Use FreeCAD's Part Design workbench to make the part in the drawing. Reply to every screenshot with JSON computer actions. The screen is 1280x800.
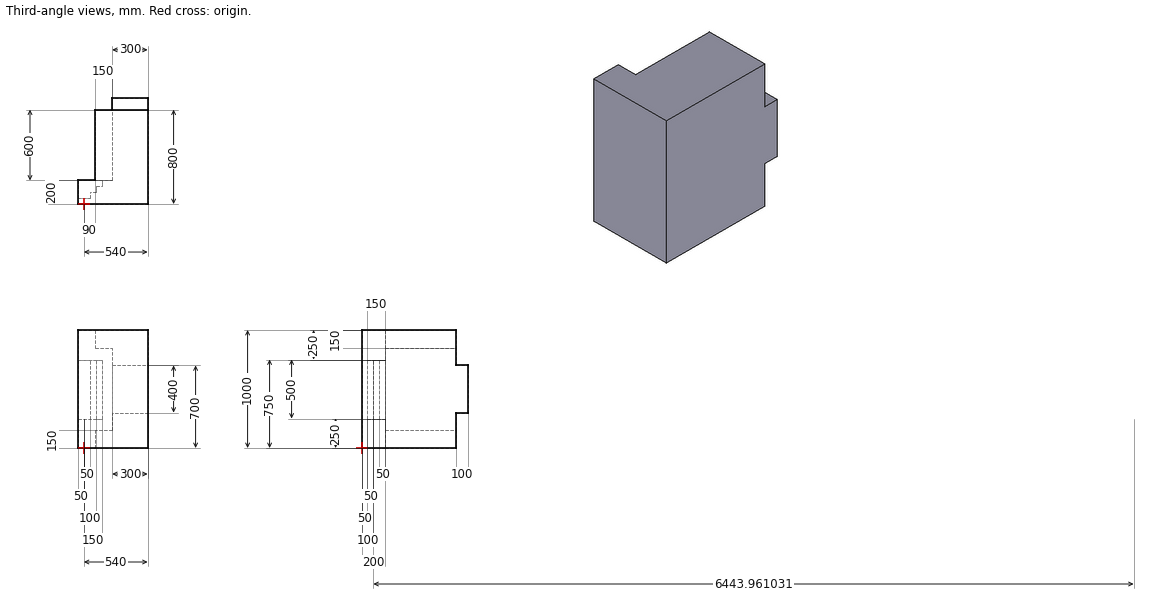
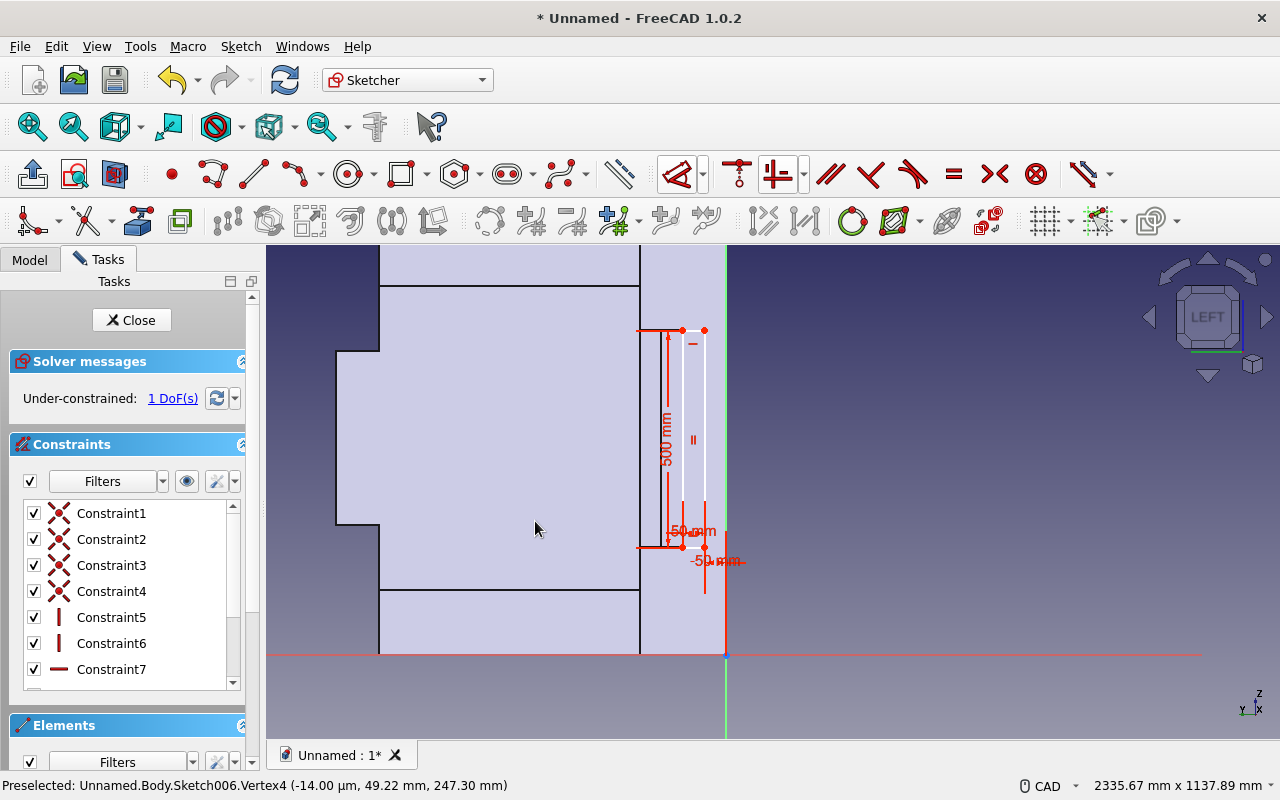
{"action": "left_click", "coordinate": [683, 331]}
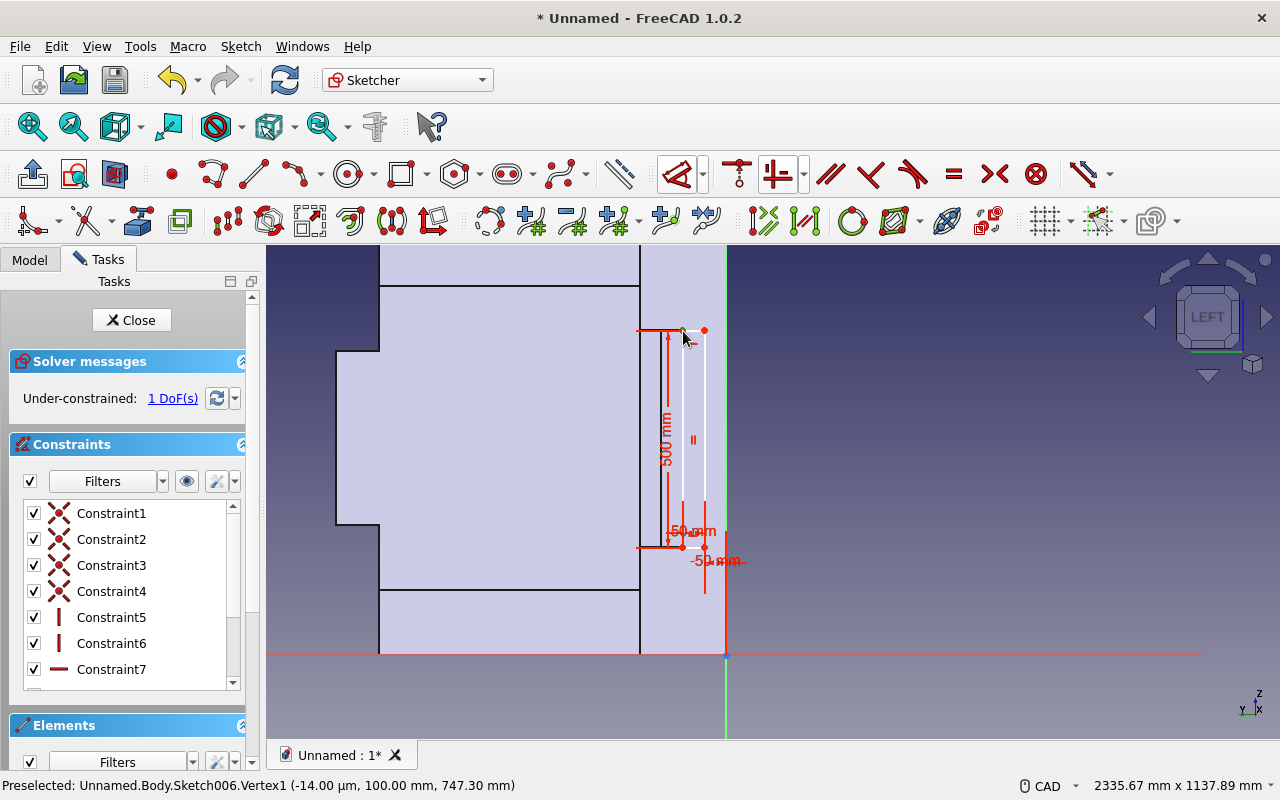
{"action": "left_click", "coordinate": [702, 174]}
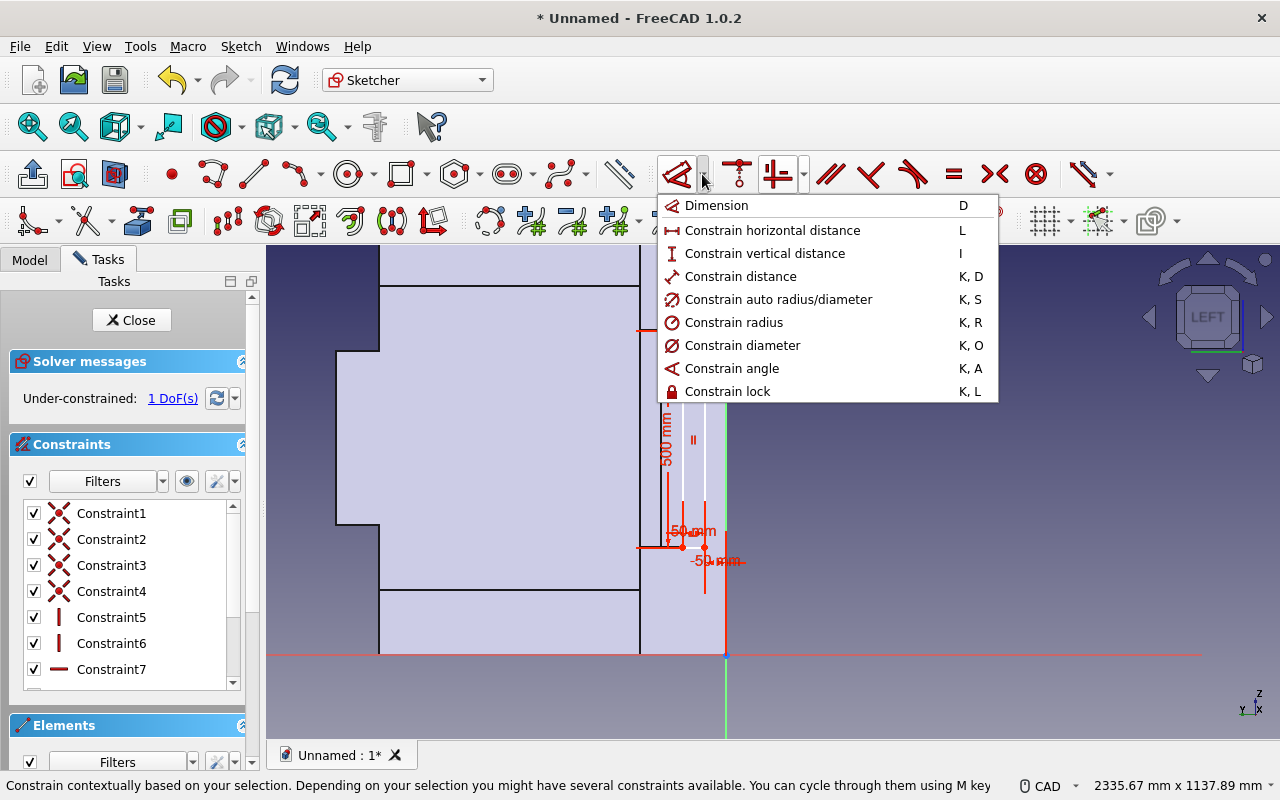
{"action": "left_click", "coordinate": [828, 254]}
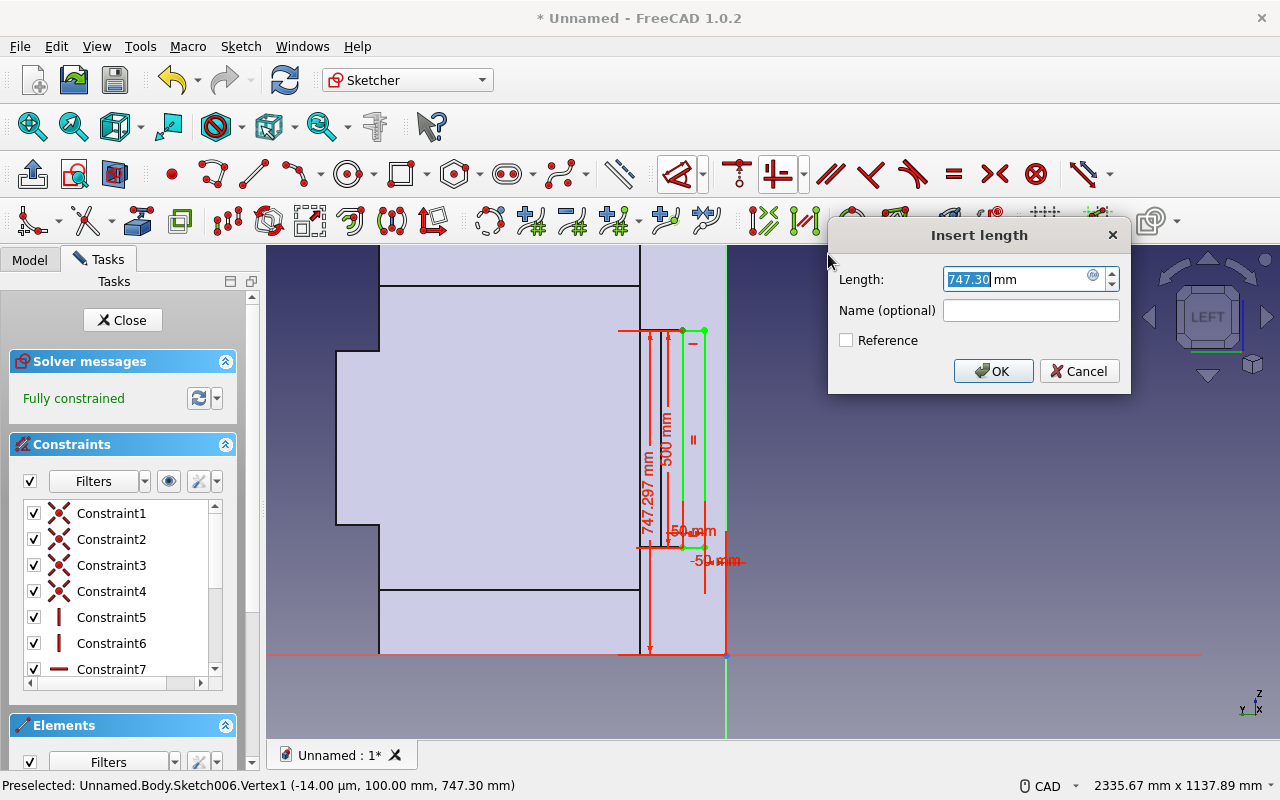
{"action": "type", "text": "750"}
{"action": "key", "text": "Return"}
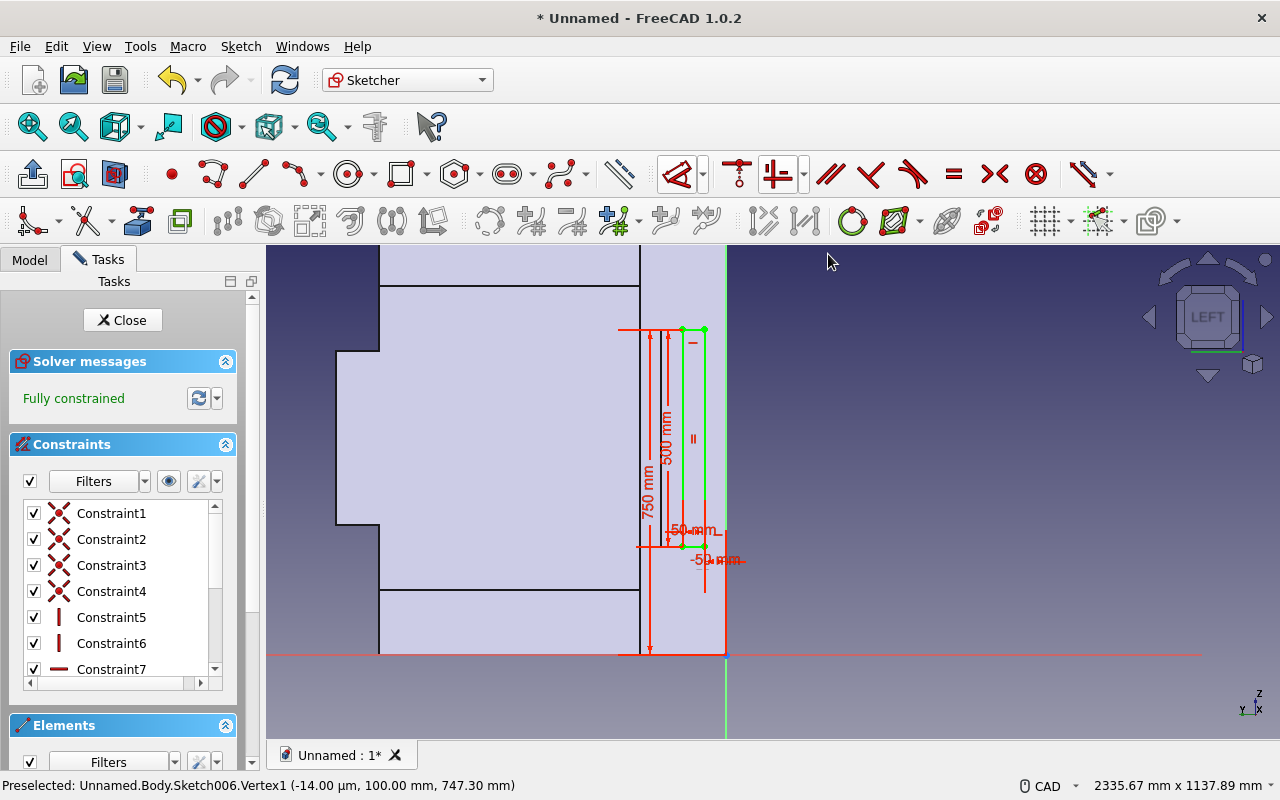
{"action": "left_click", "coordinate": [123, 320]}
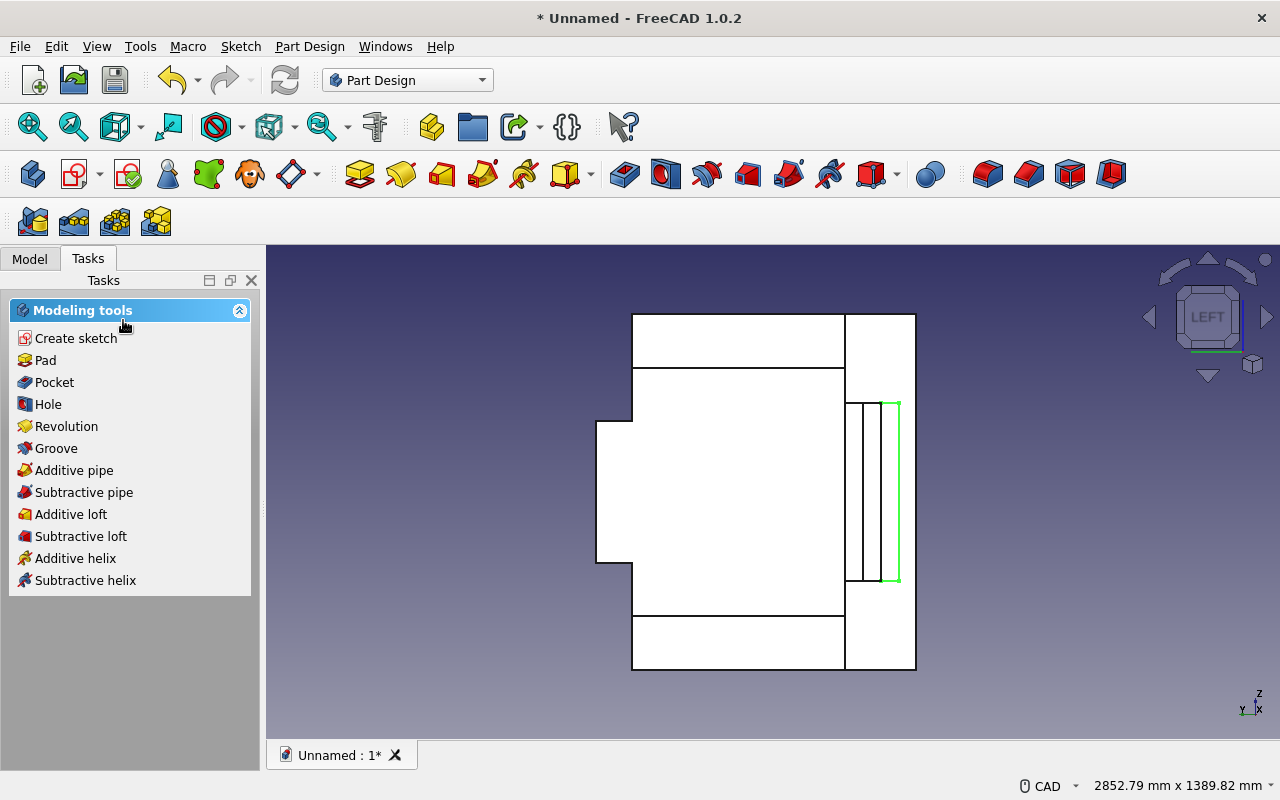
{"action": "left_click", "coordinate": [625, 174]}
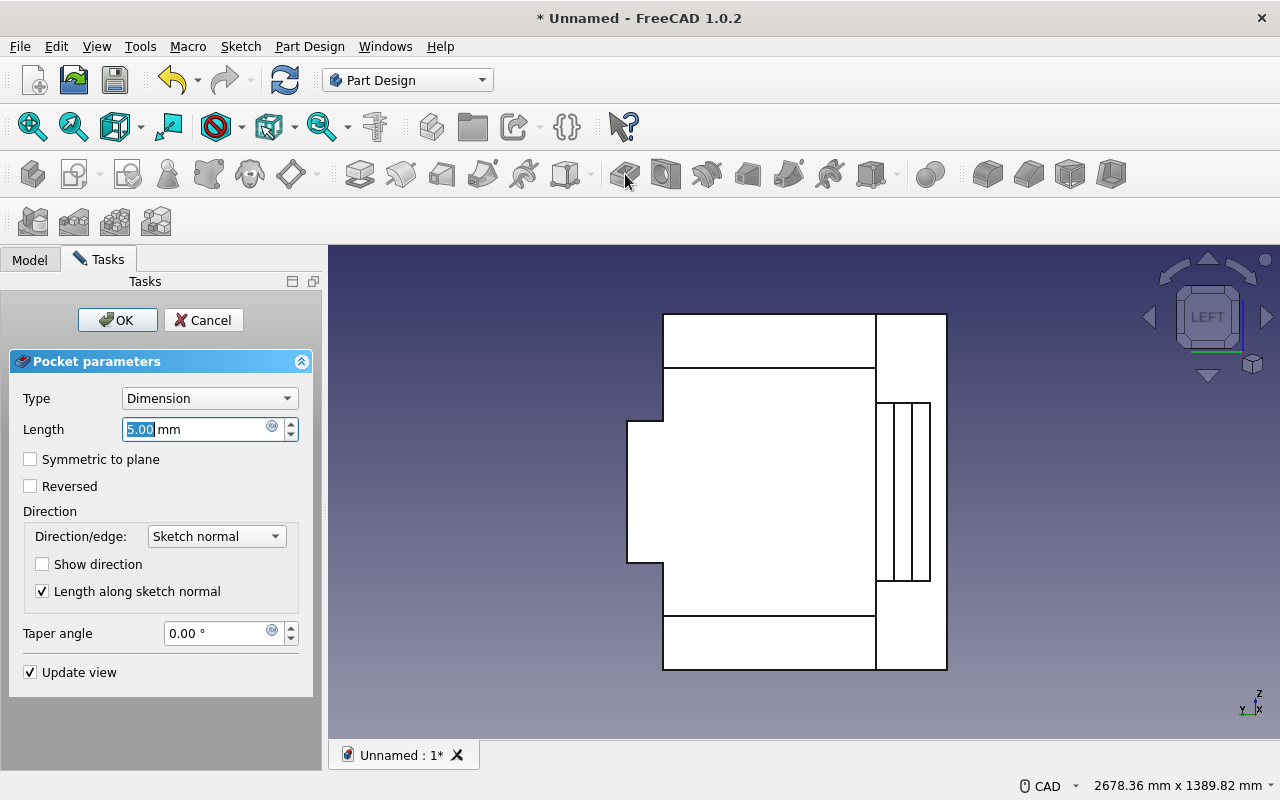
{"action": "type", "text": "50"}
{"action": "key", "text": "Tab"}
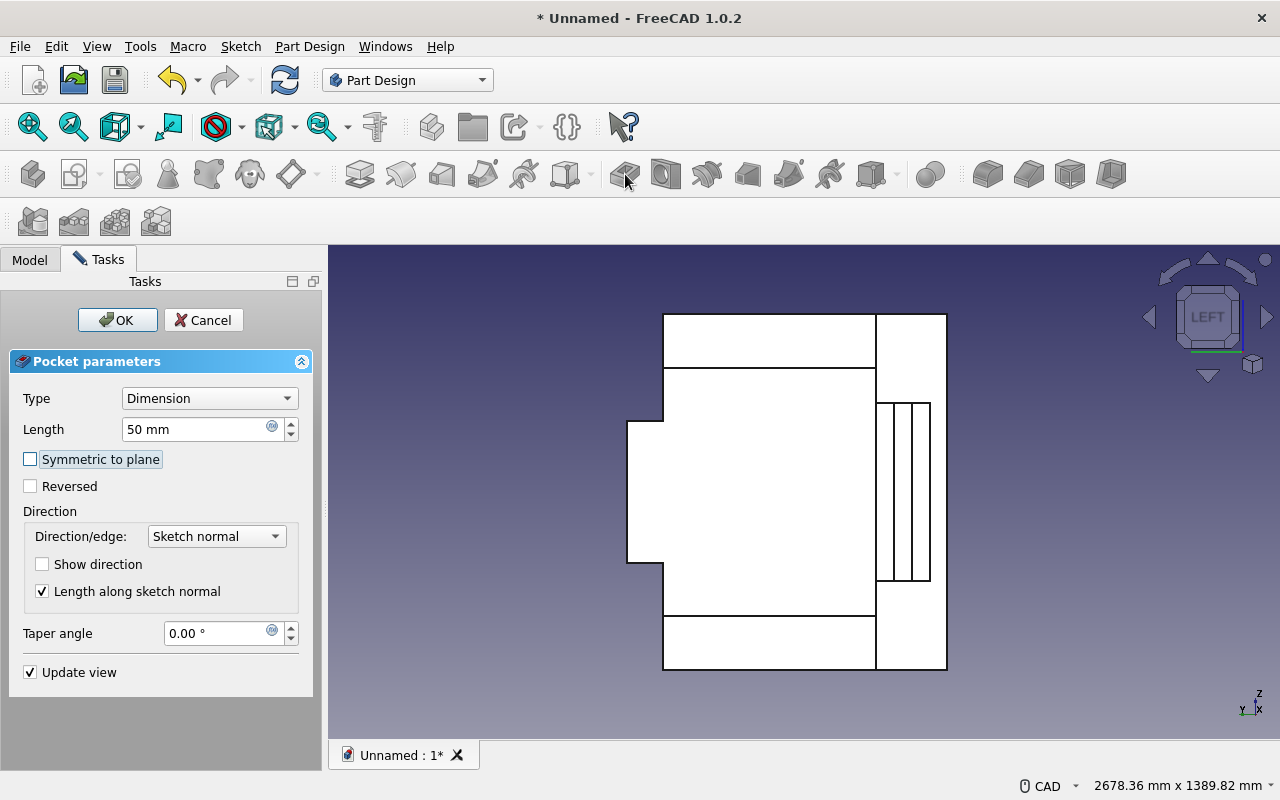
{"action": "left_click", "coordinate": [118, 320]}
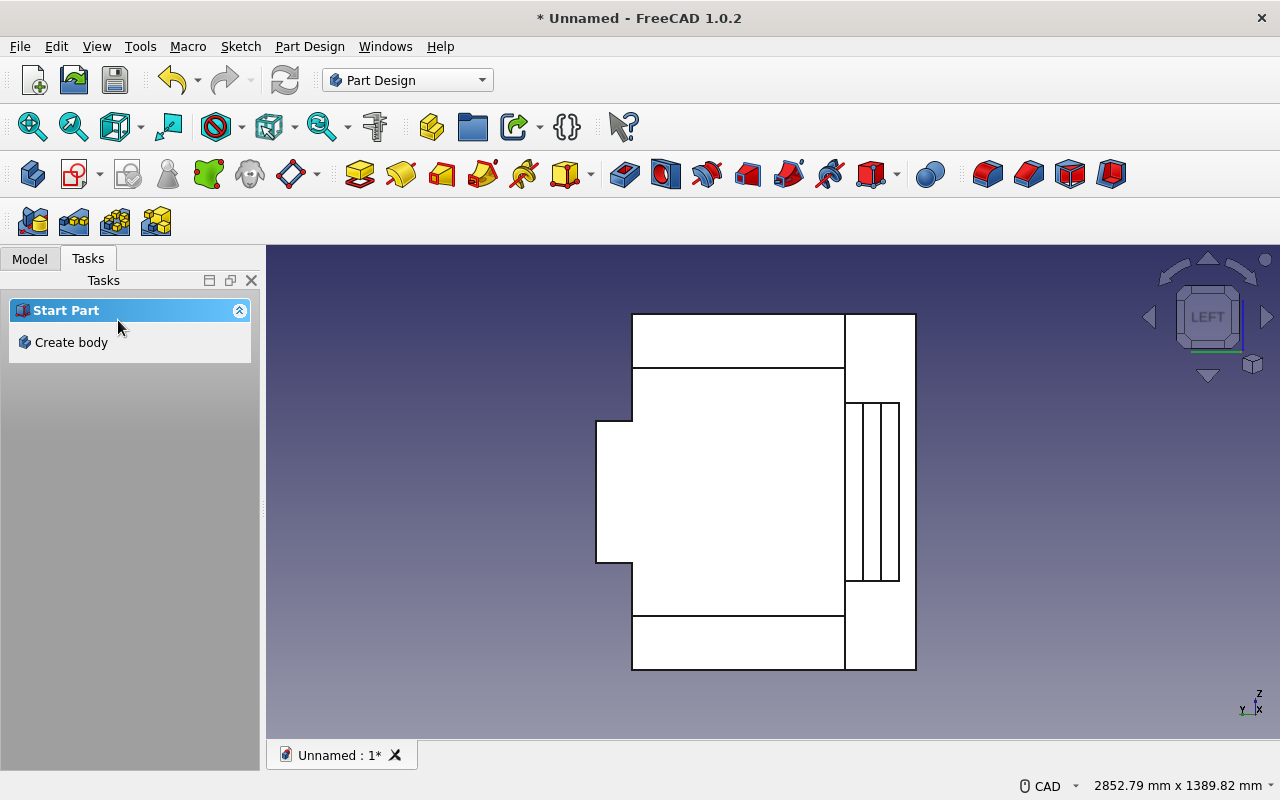
{"action": "left_click", "coordinate": [74, 174]}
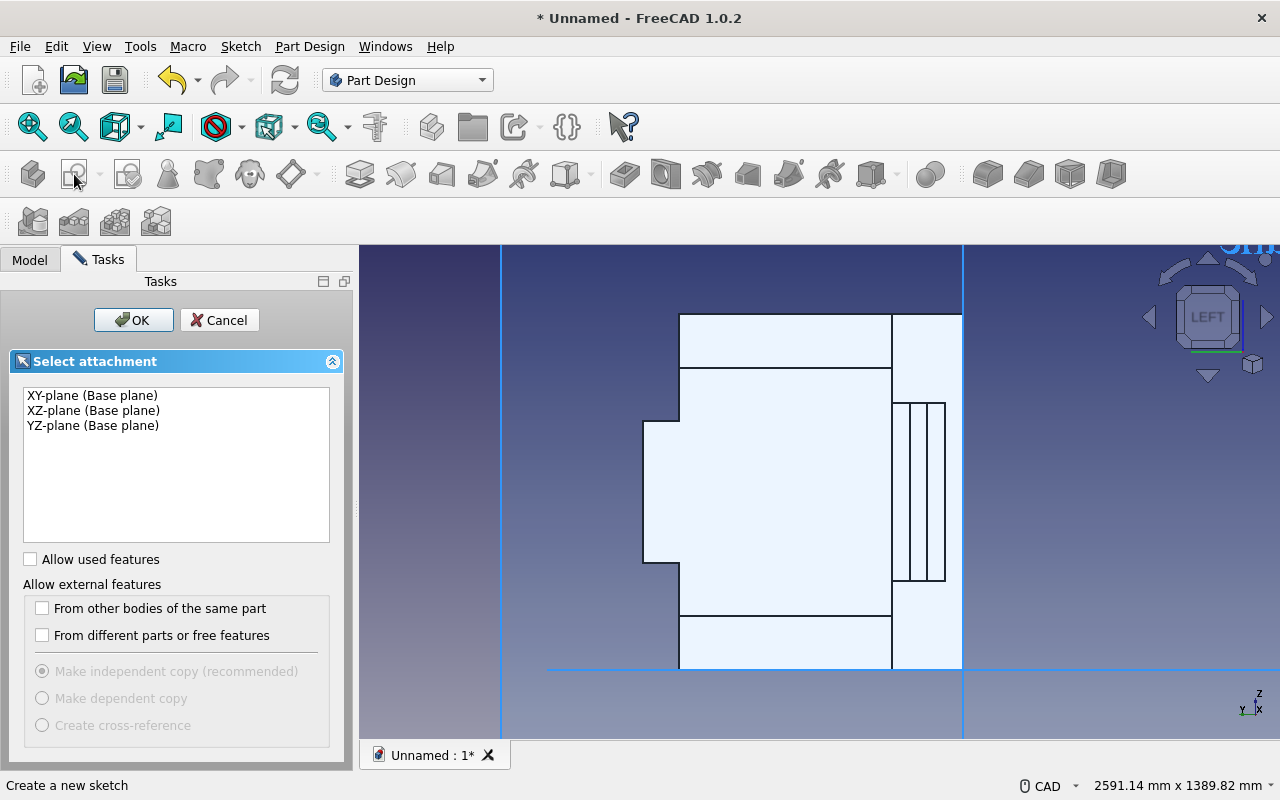
{"action": "left_click", "coordinate": [84, 426]}